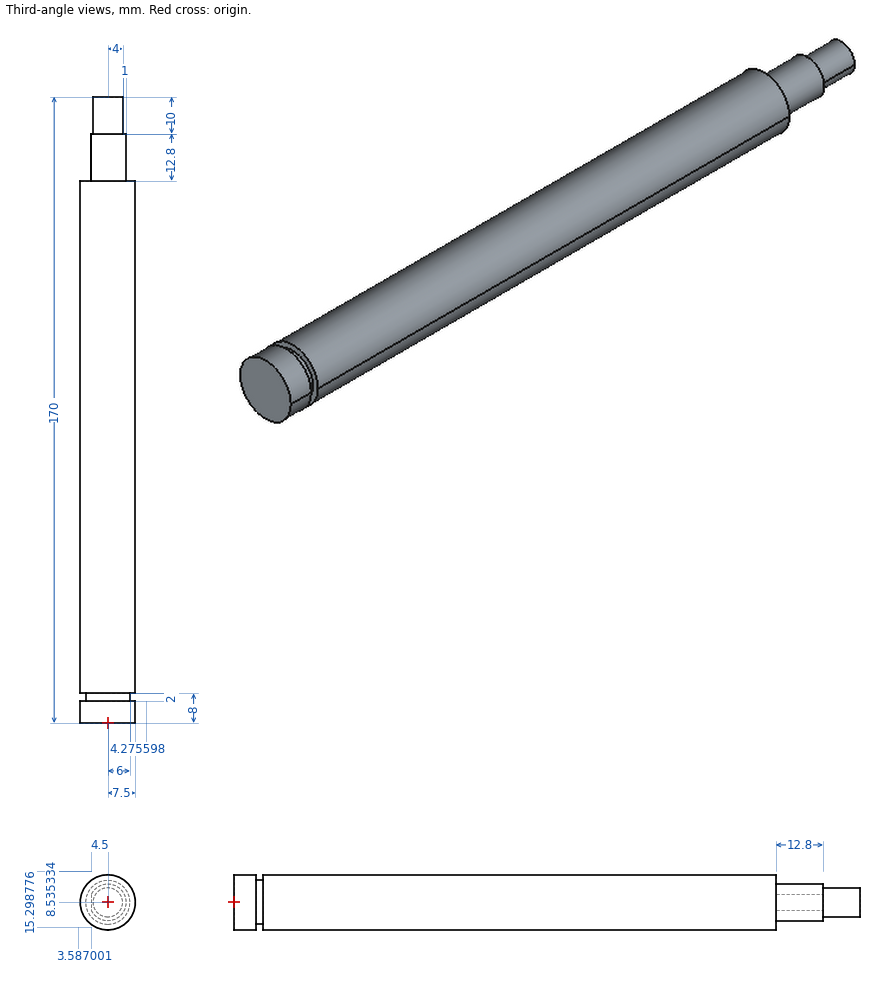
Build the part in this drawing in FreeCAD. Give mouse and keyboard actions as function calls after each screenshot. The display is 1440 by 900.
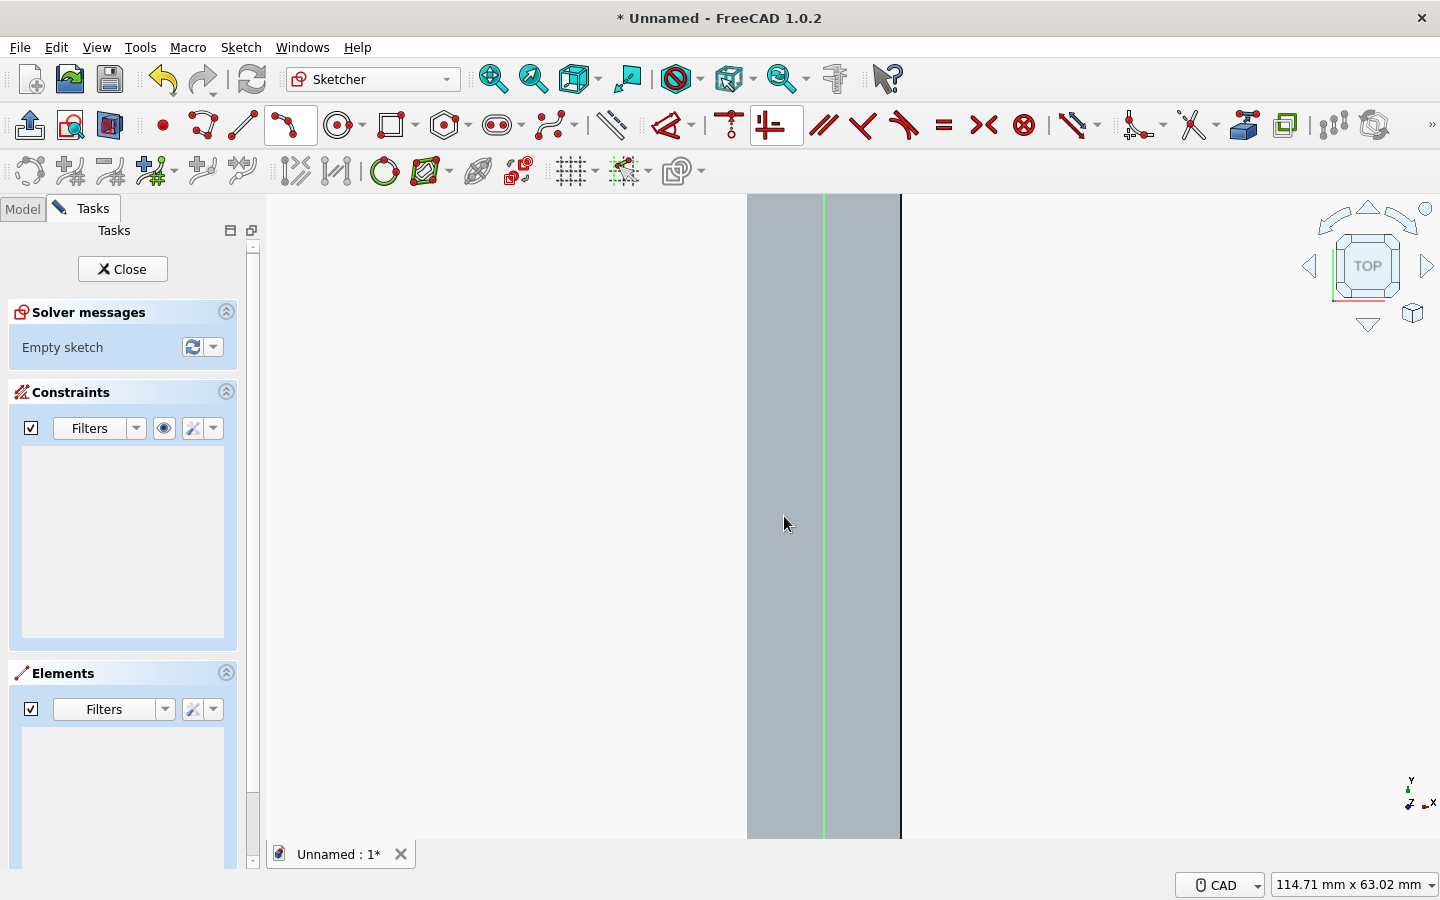
scroll(784, 516, down, 5)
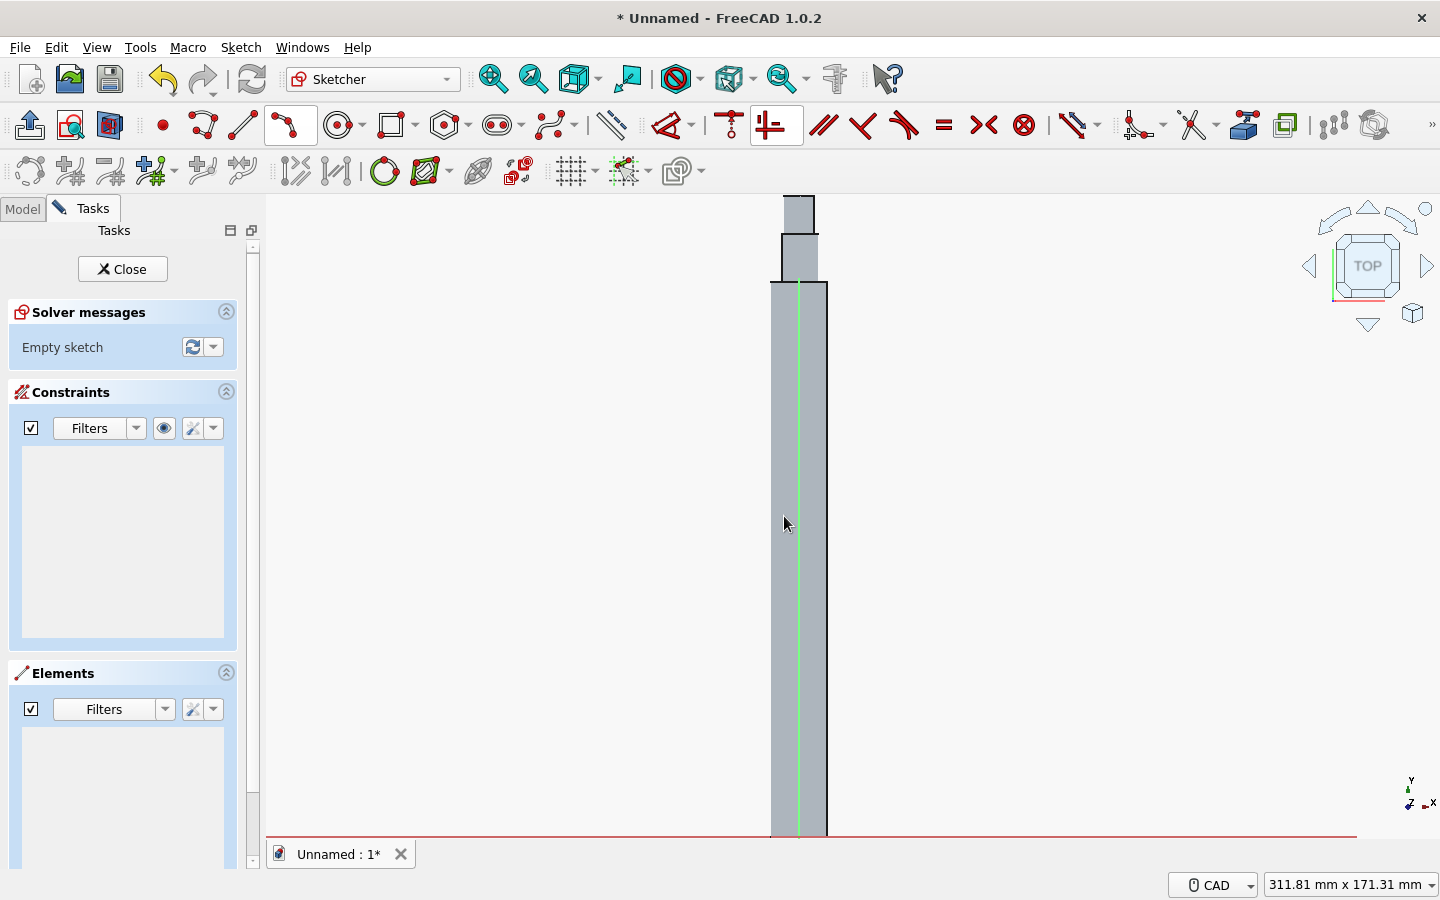
scroll(784, 516, down, 5)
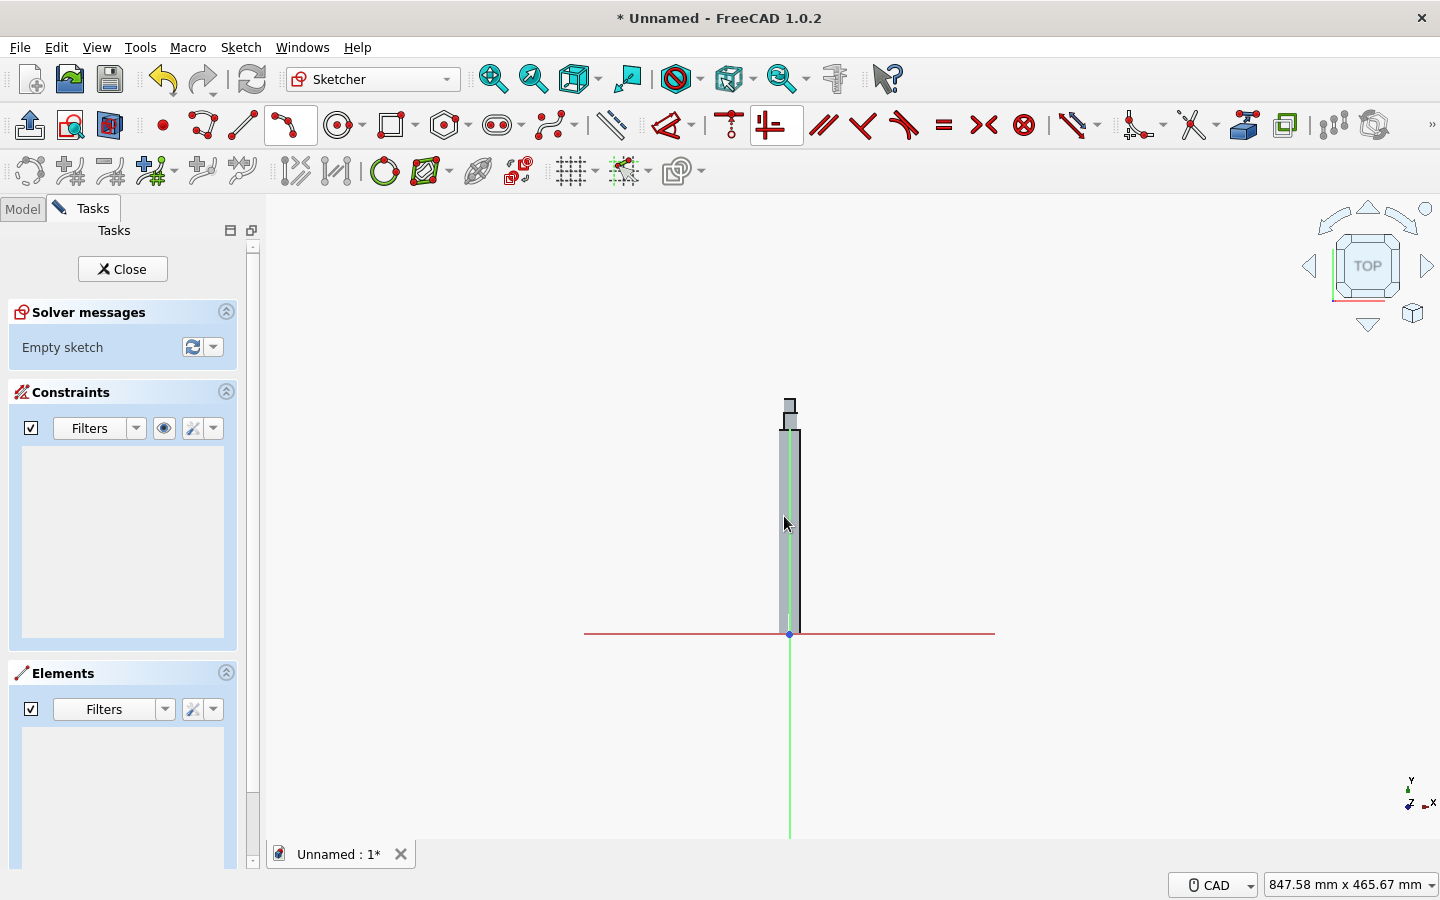
scroll(798, 635, up, 15)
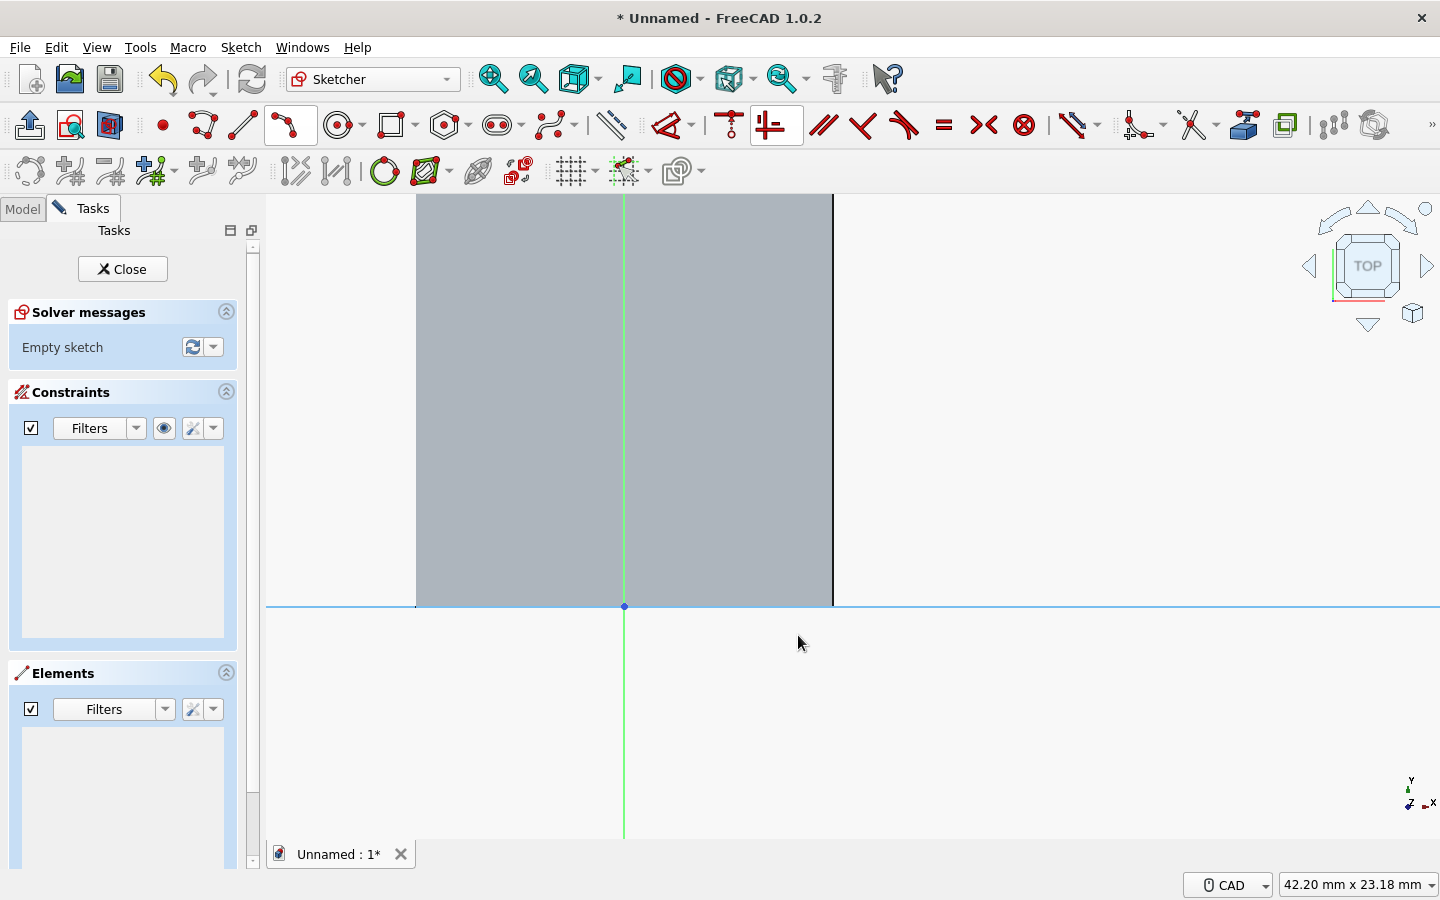
scroll(746, 469, up, 3)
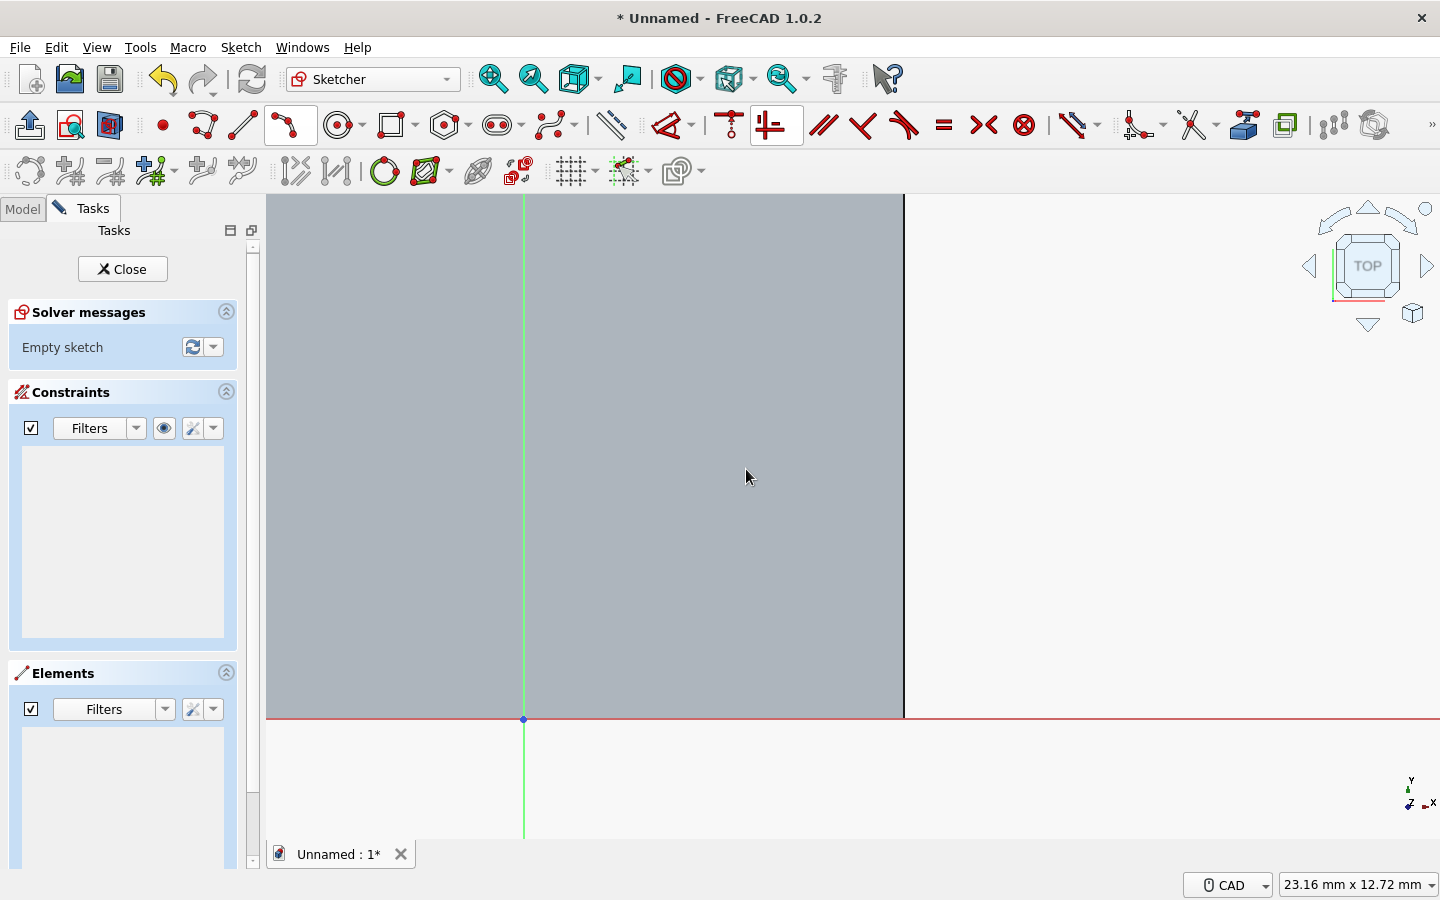
click(392, 126)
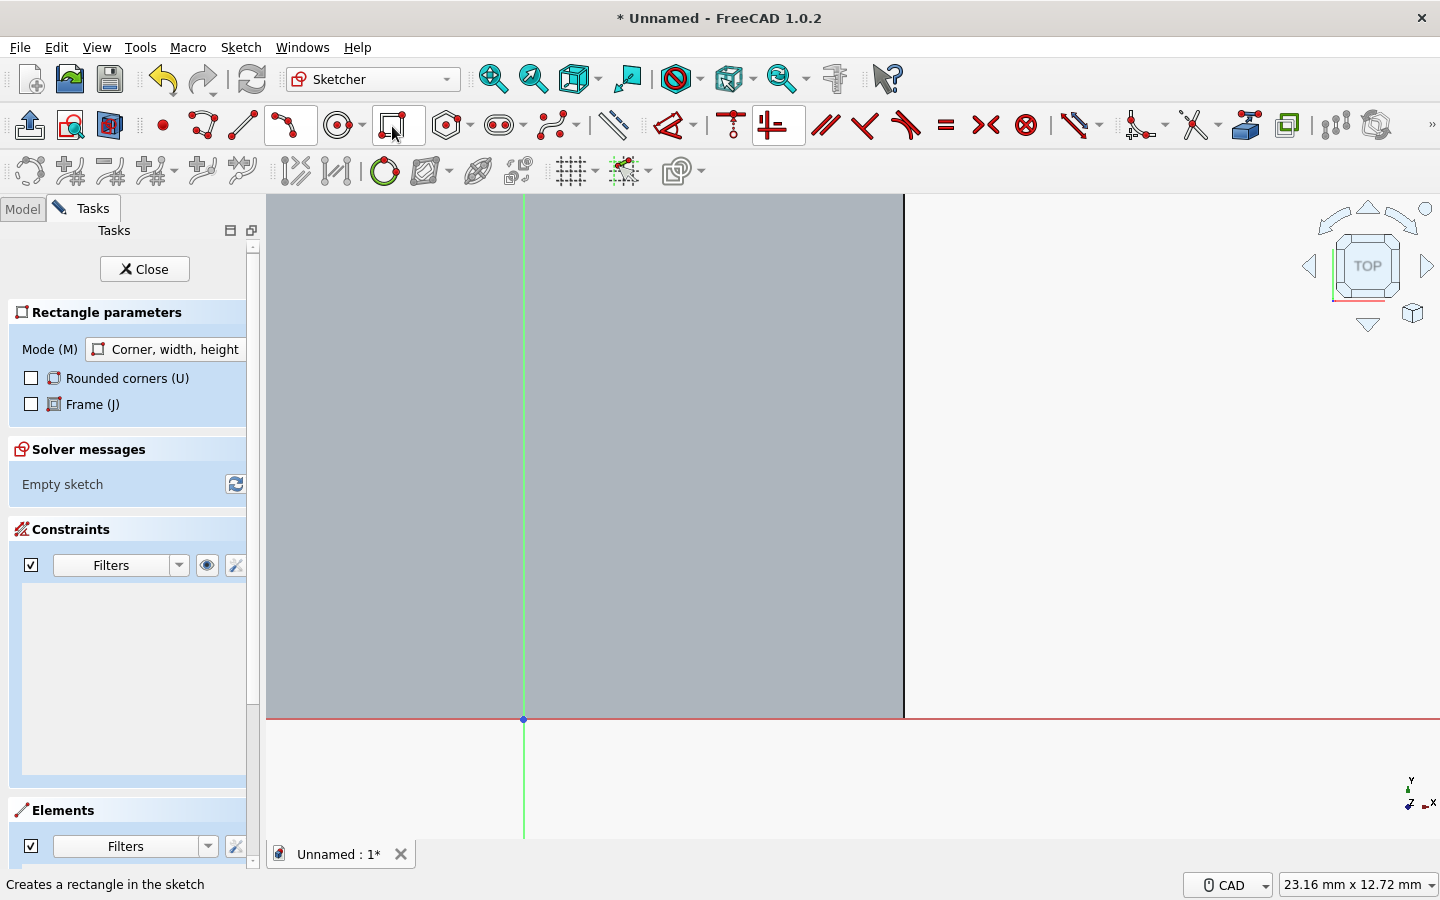
click(828, 314)
click(1045, 415)
key(Escape)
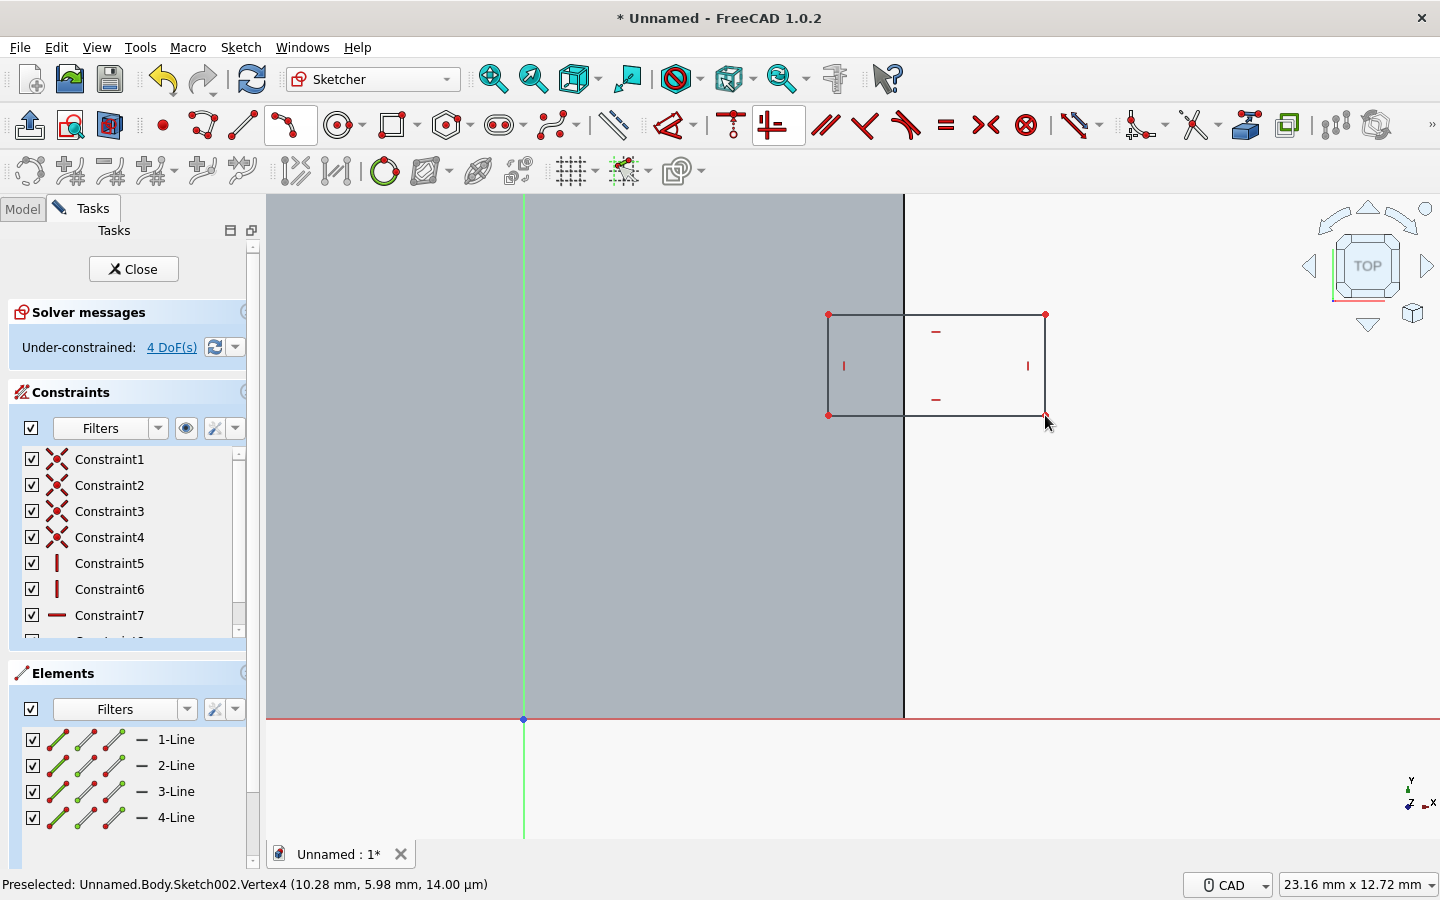
click(668, 126)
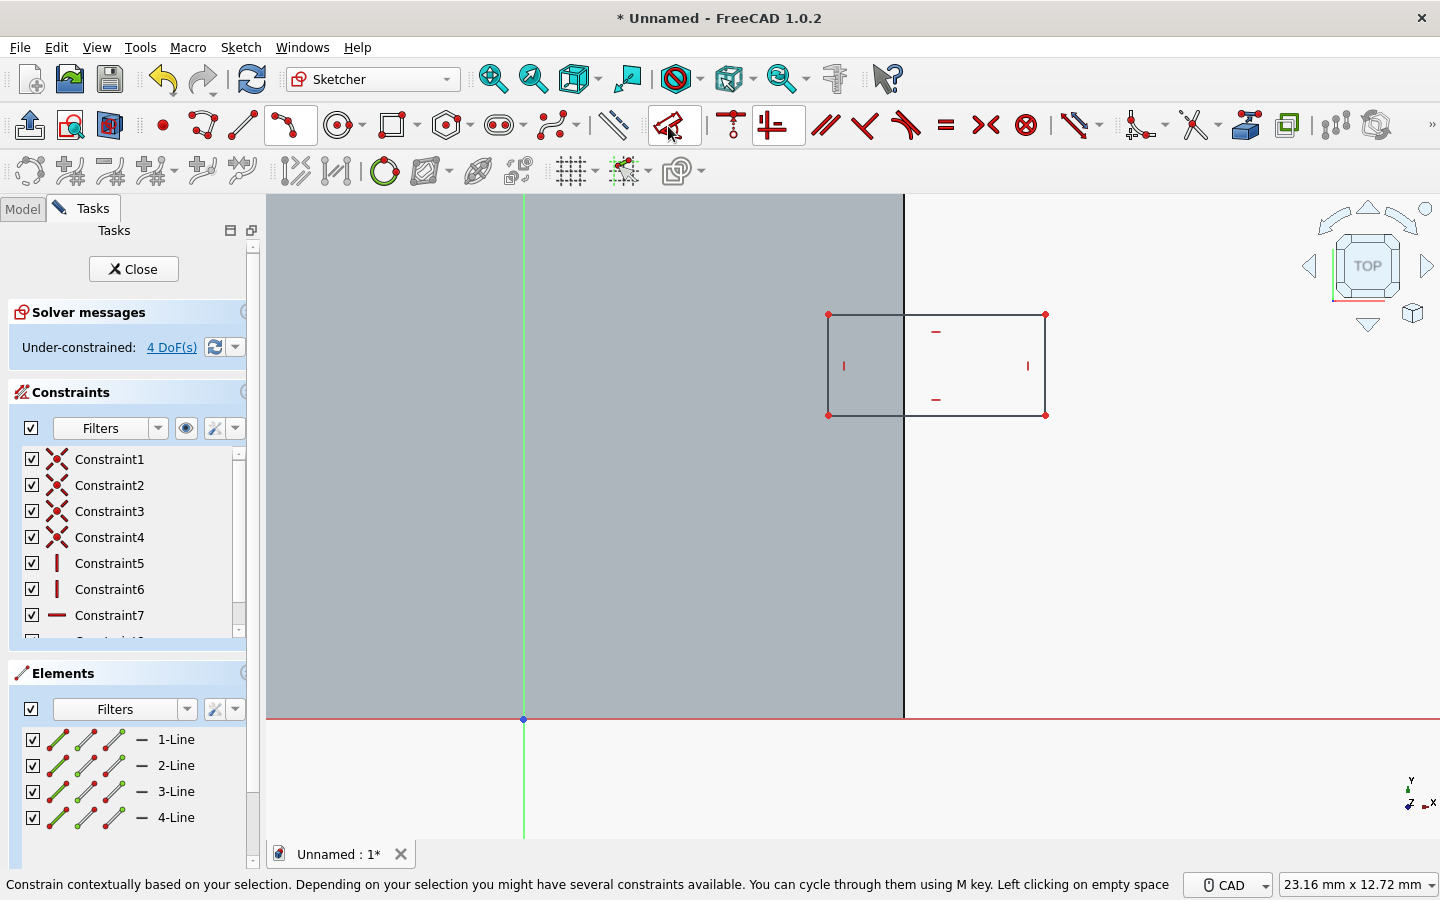
click(828, 345)
click(862, 366)